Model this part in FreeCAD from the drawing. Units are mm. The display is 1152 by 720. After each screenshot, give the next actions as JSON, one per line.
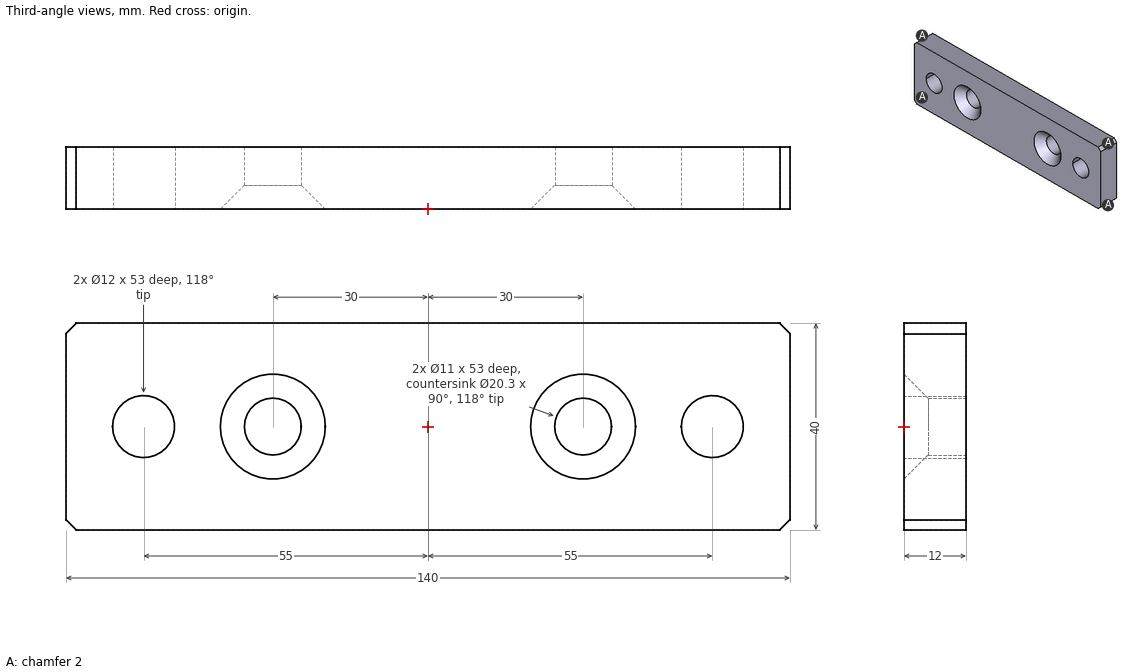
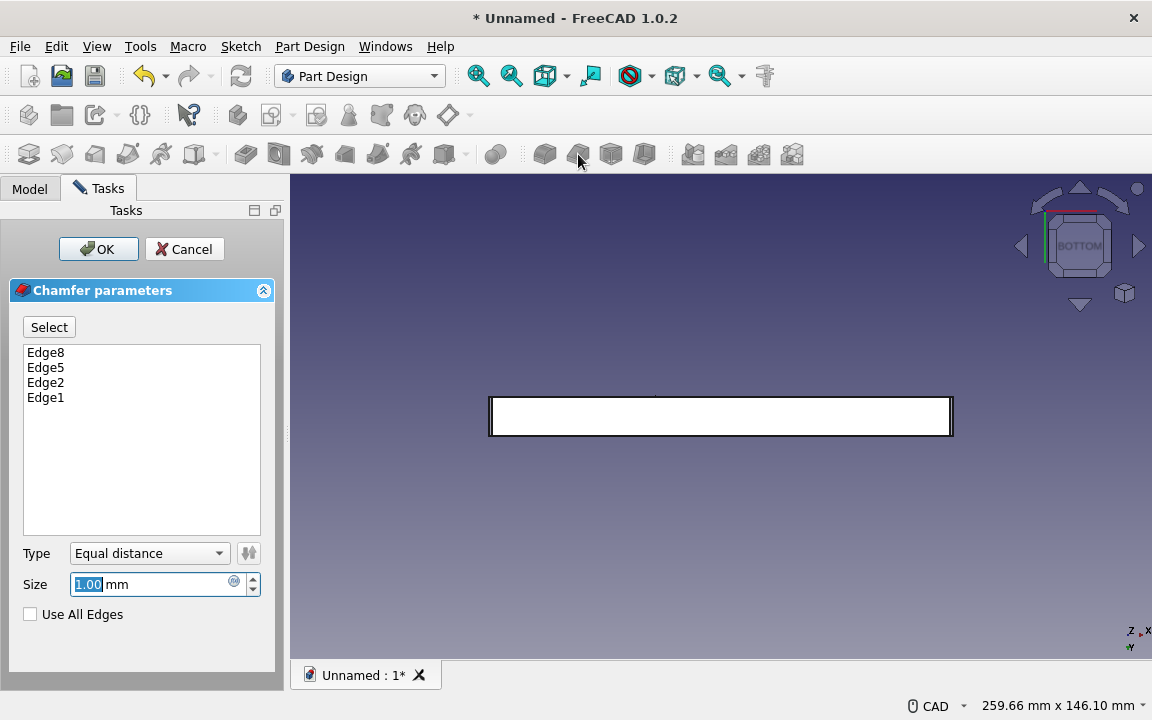
{"action": "type", "text": "2"}
{"action": "key", "text": "Tab"}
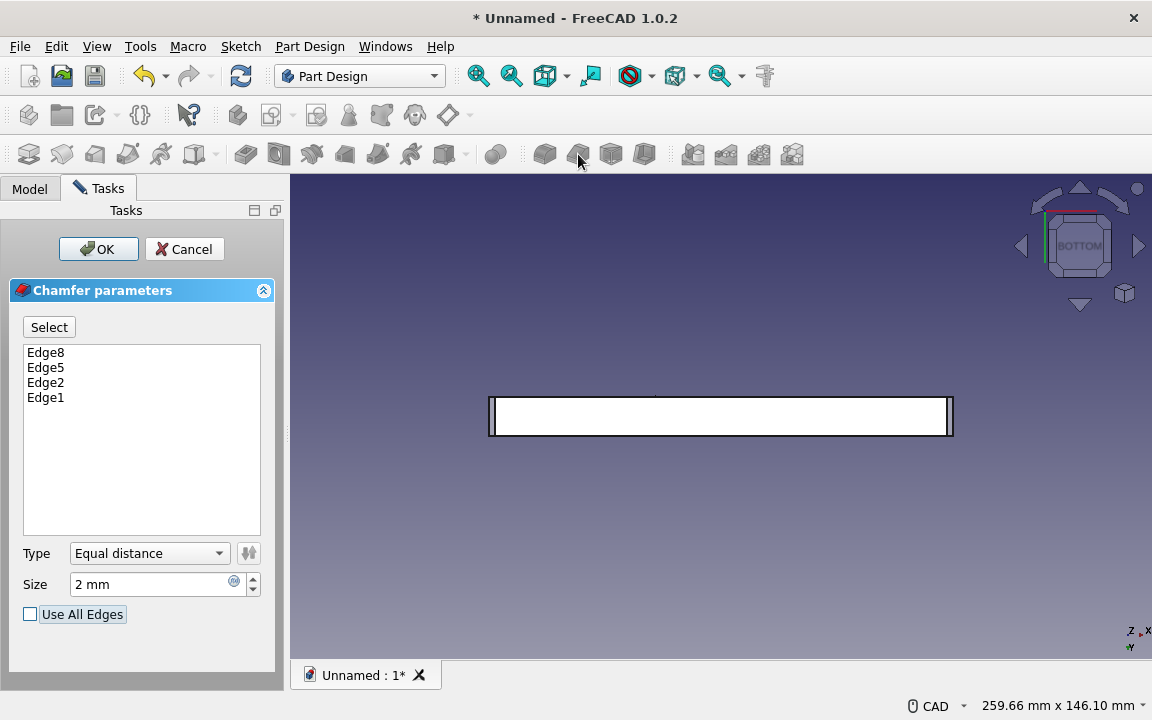
{"action": "left_click", "coordinate": [99, 249]}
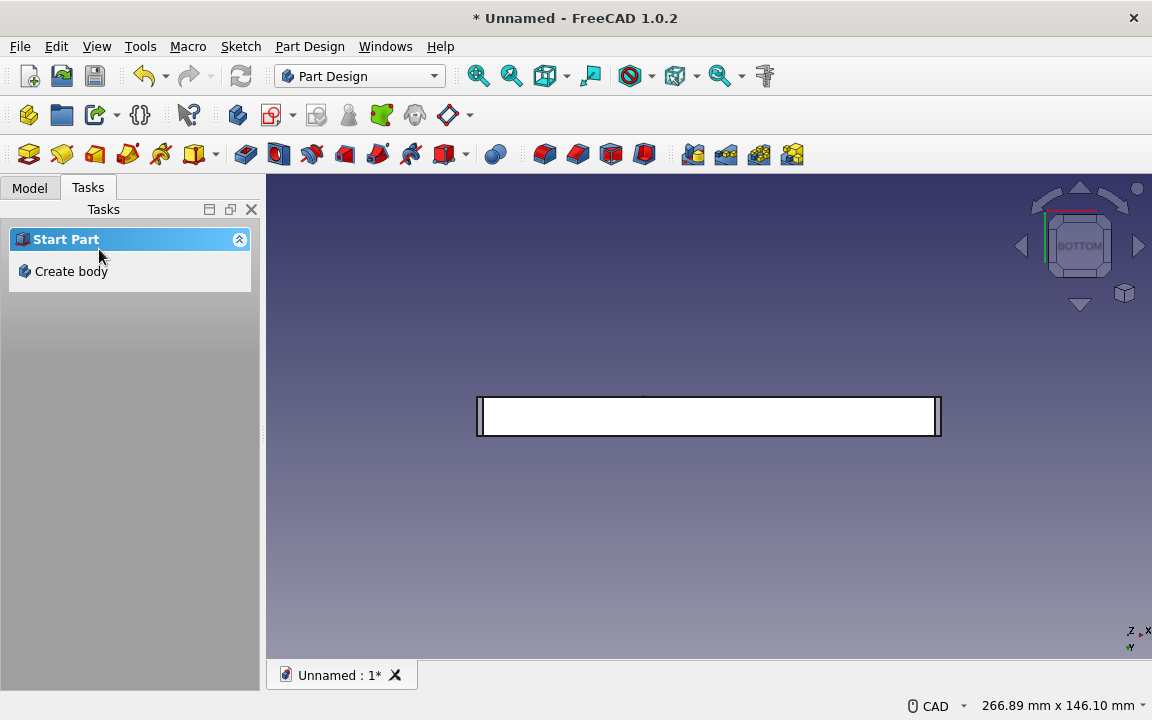
{"action": "key", "text": "0"}